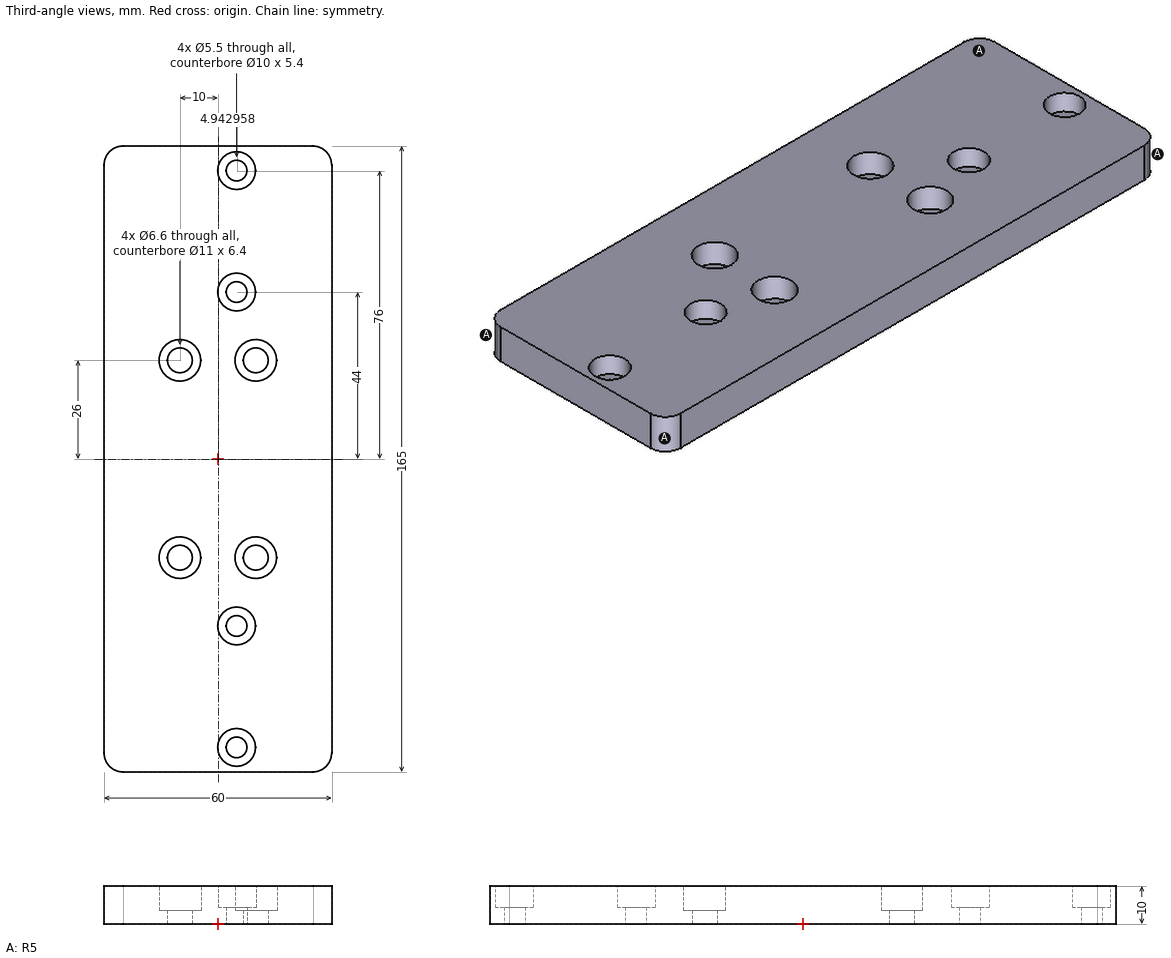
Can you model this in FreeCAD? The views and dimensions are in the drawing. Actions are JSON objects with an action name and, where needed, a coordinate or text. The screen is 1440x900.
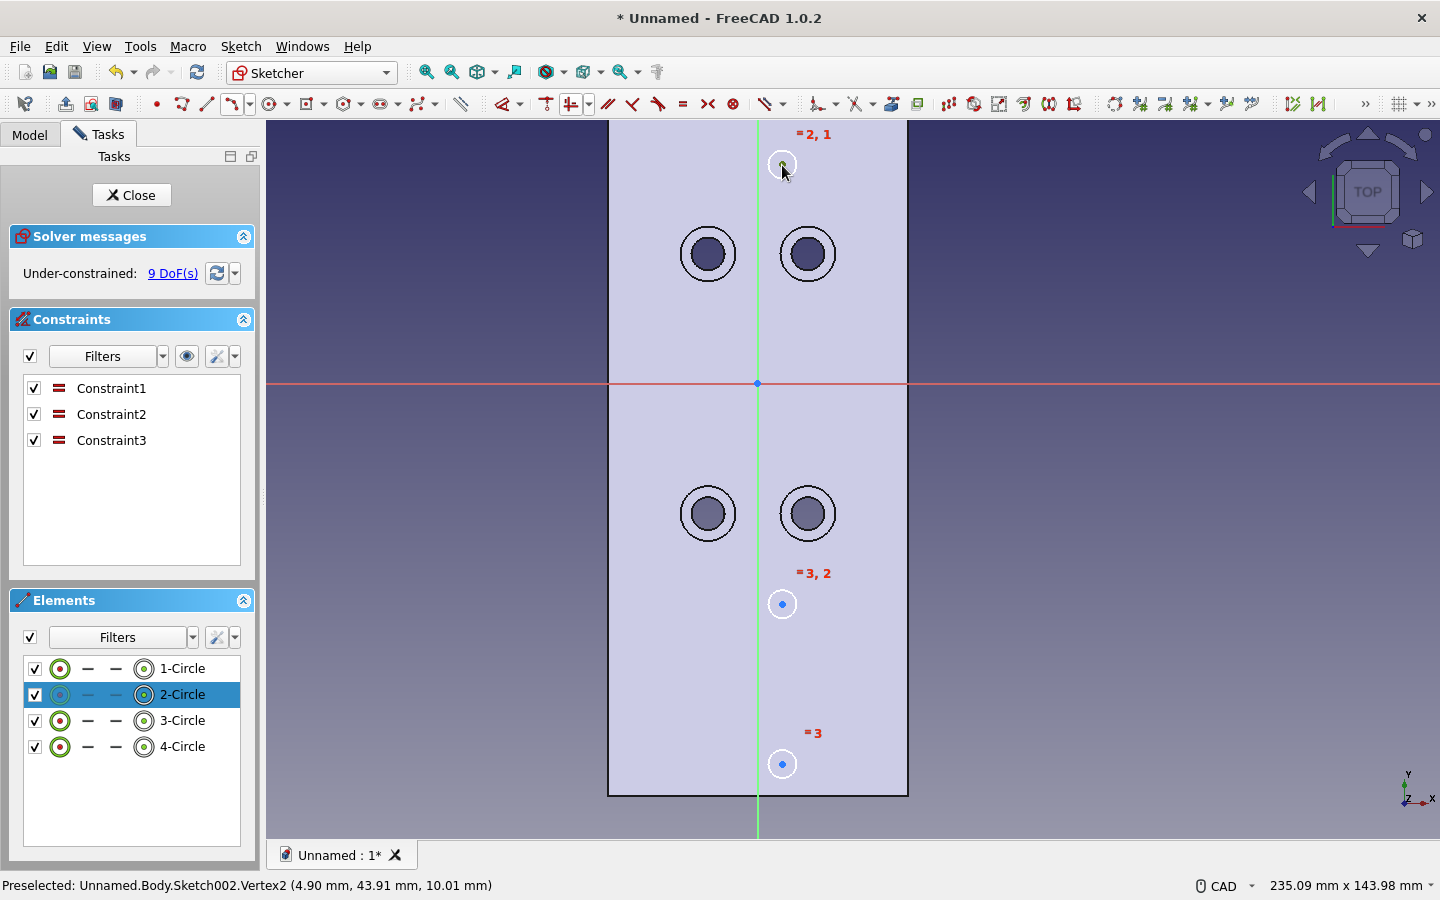
{"action": "left_click", "coordinate": [782, 604]}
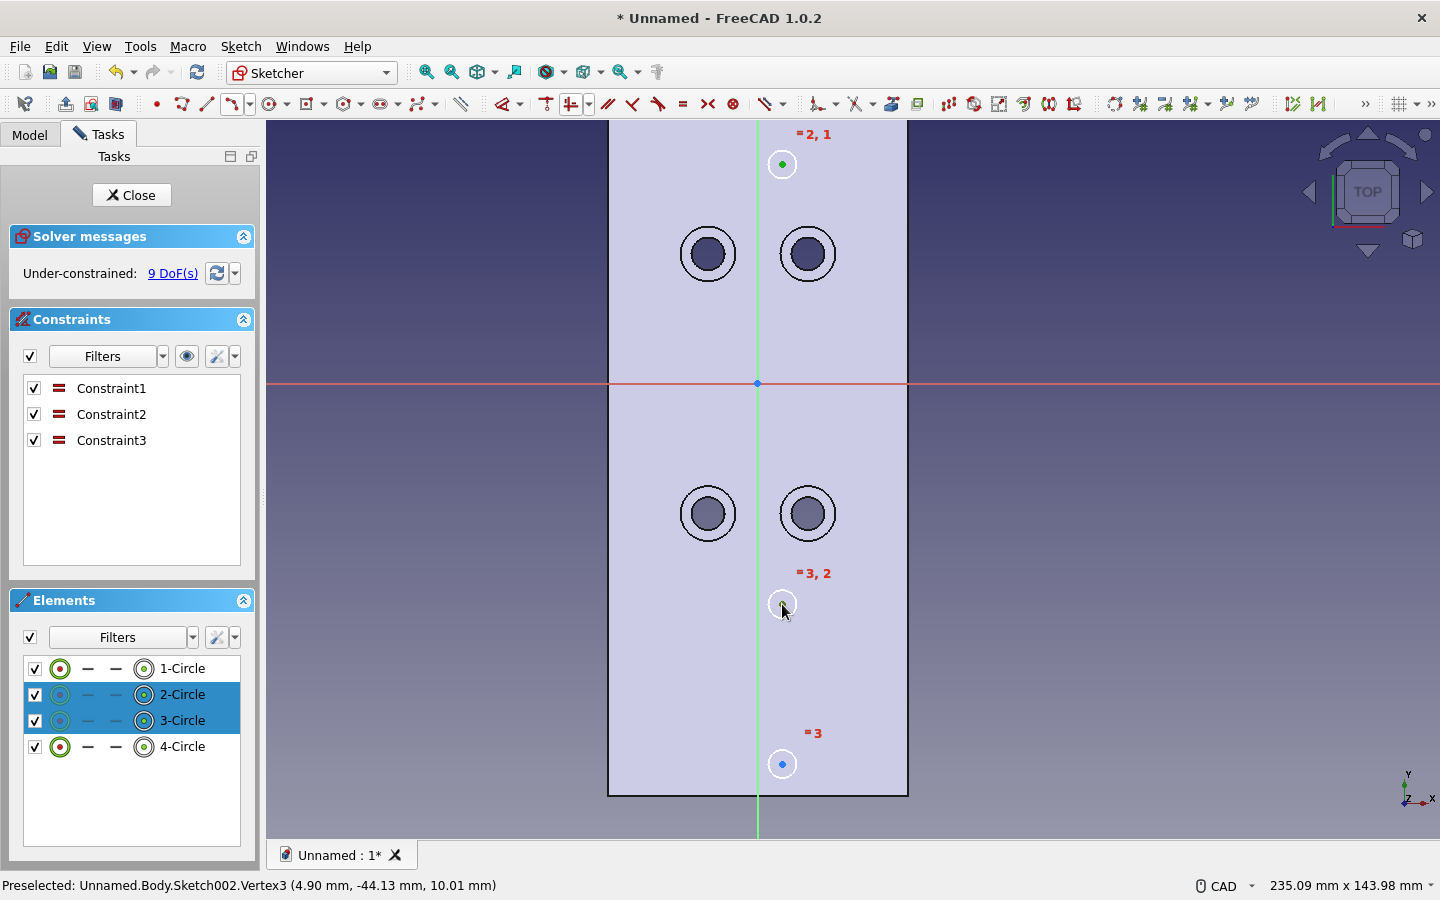
{"action": "left_click", "coordinate": [364, 384]}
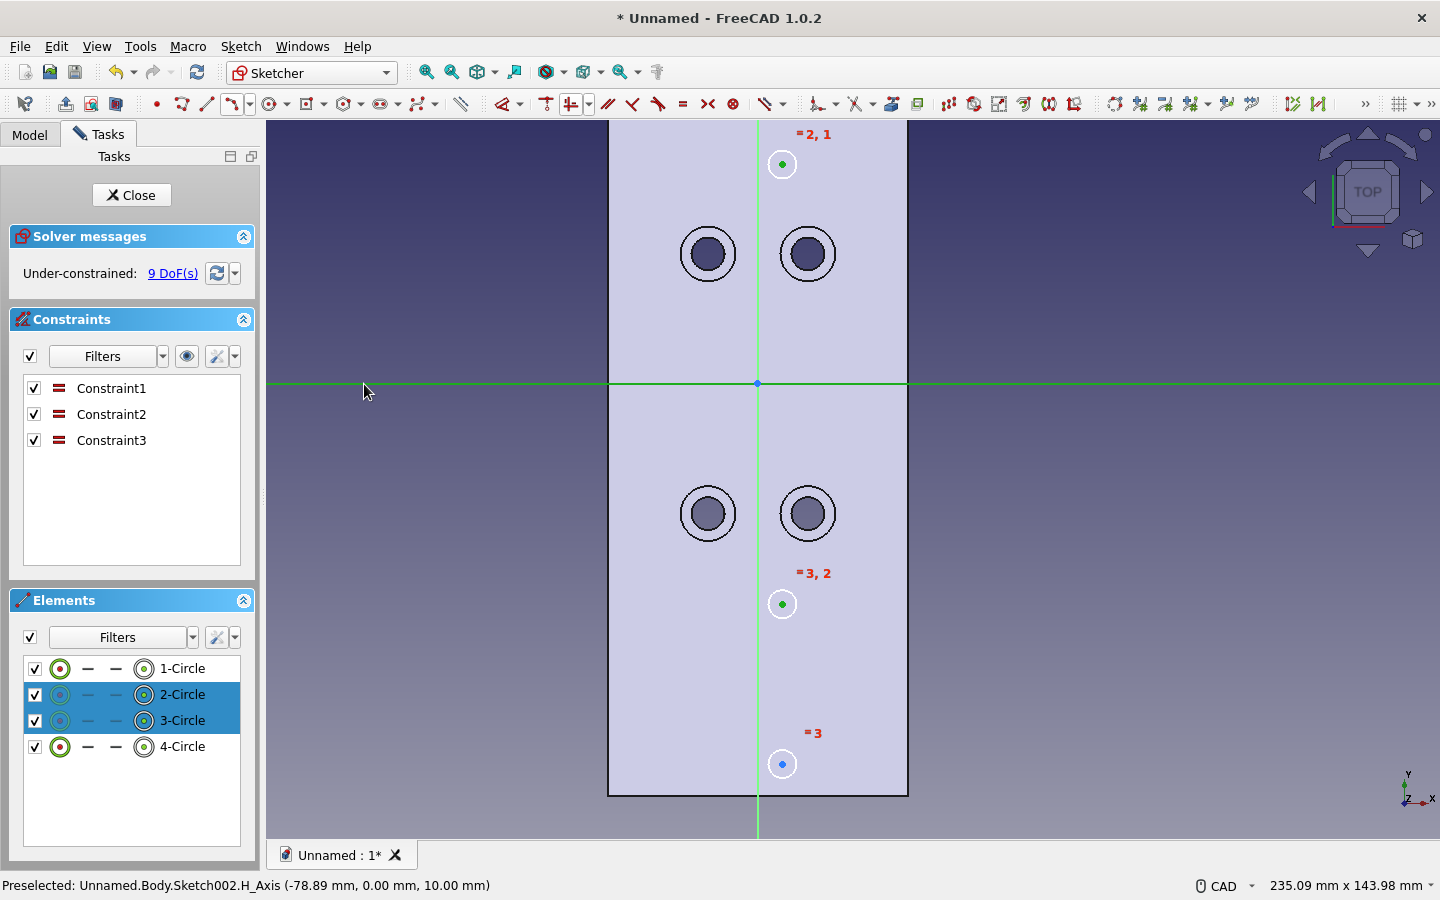
{"action": "left_click", "coordinate": [708, 104]}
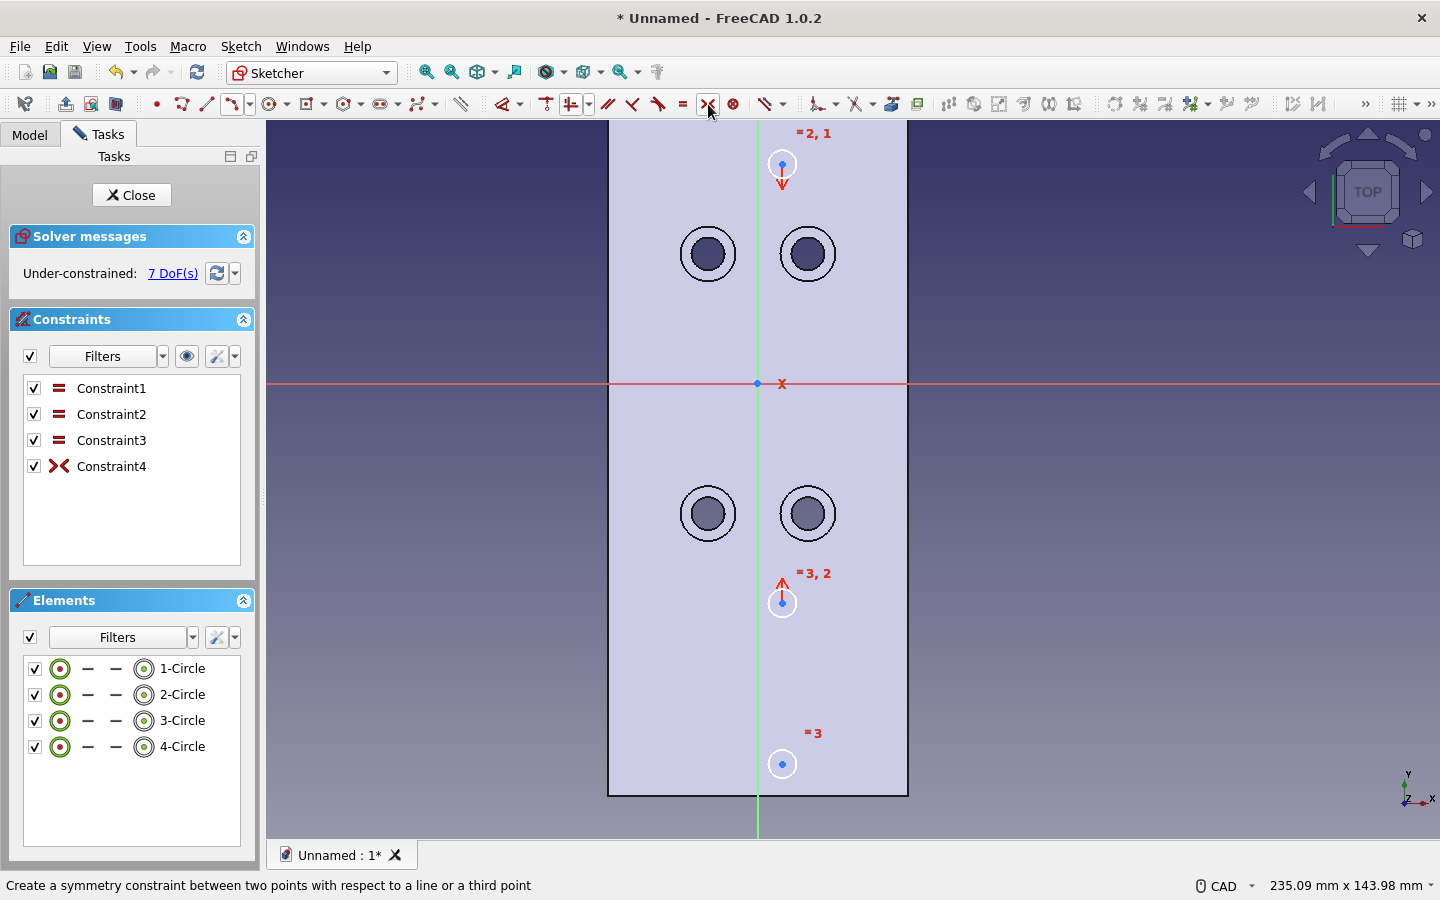
{"action": "scroll", "coordinate": [793, 596], "scroll_direction": "down", "scroll_amount": 3}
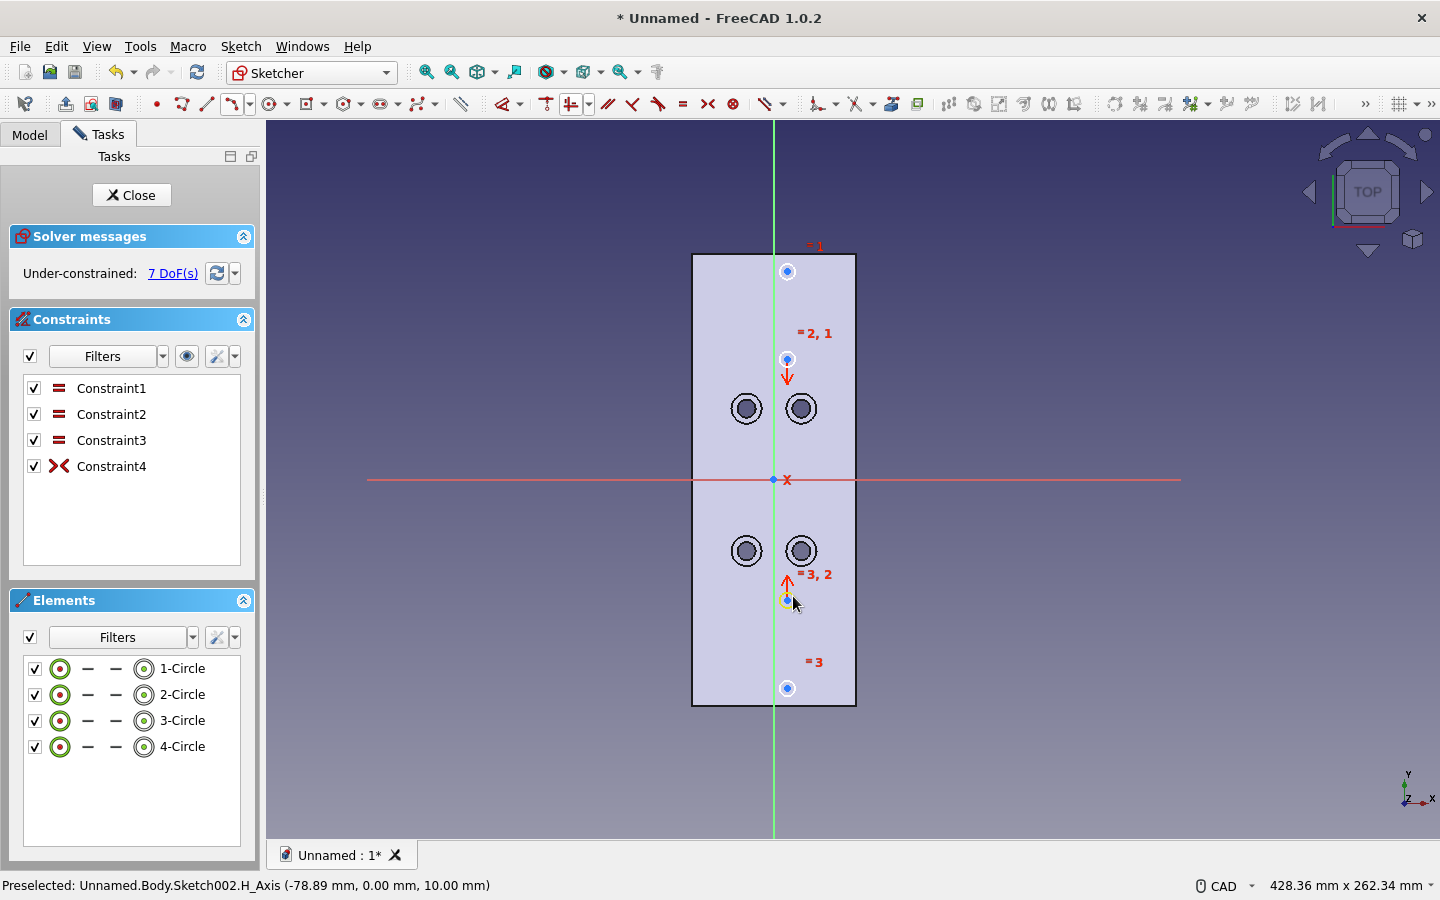
{"action": "left_click", "coordinate": [787, 272]}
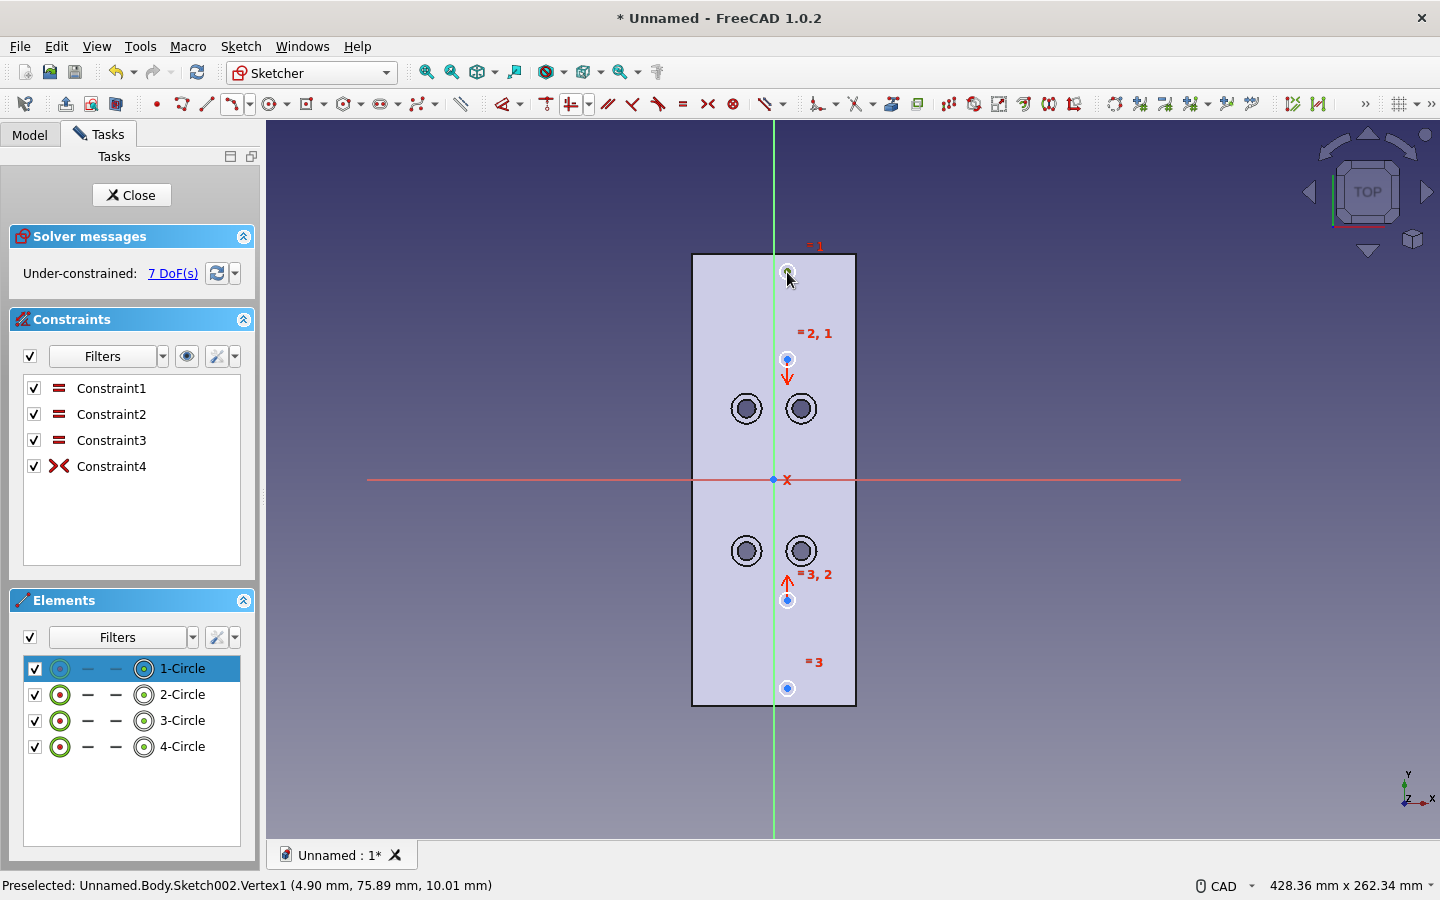
{"action": "left_click", "coordinate": [787, 689]}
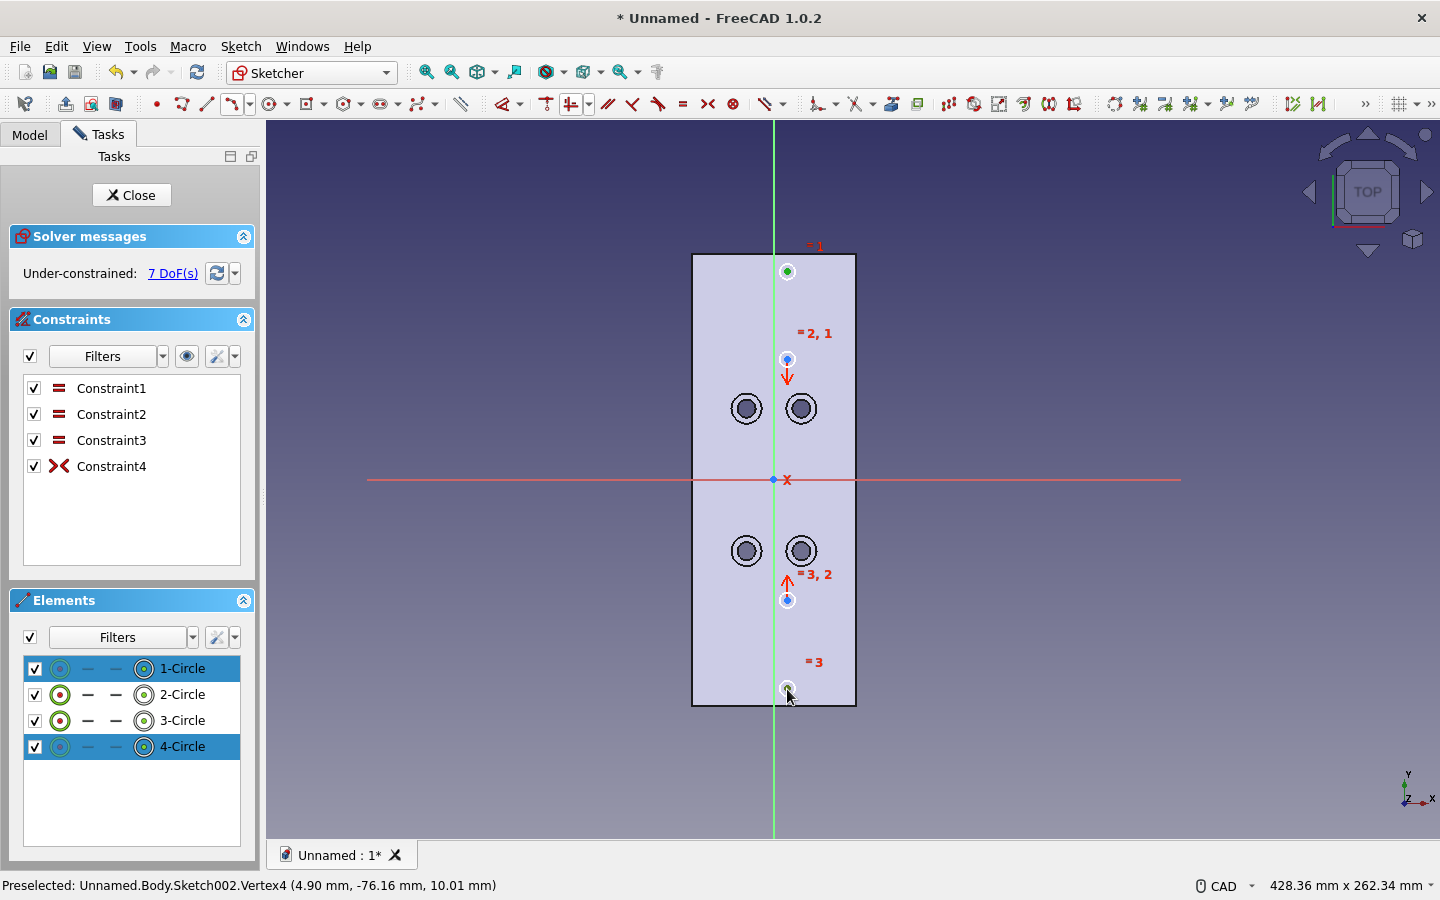
{"action": "left_click", "coordinate": [364, 480]}